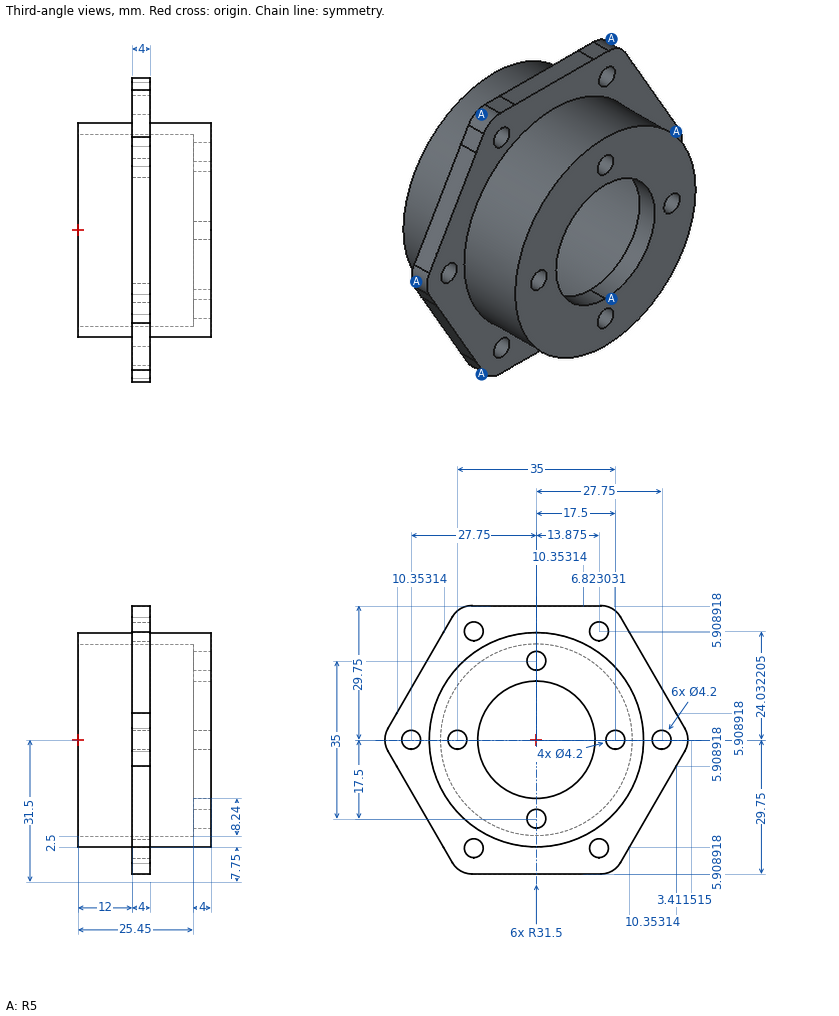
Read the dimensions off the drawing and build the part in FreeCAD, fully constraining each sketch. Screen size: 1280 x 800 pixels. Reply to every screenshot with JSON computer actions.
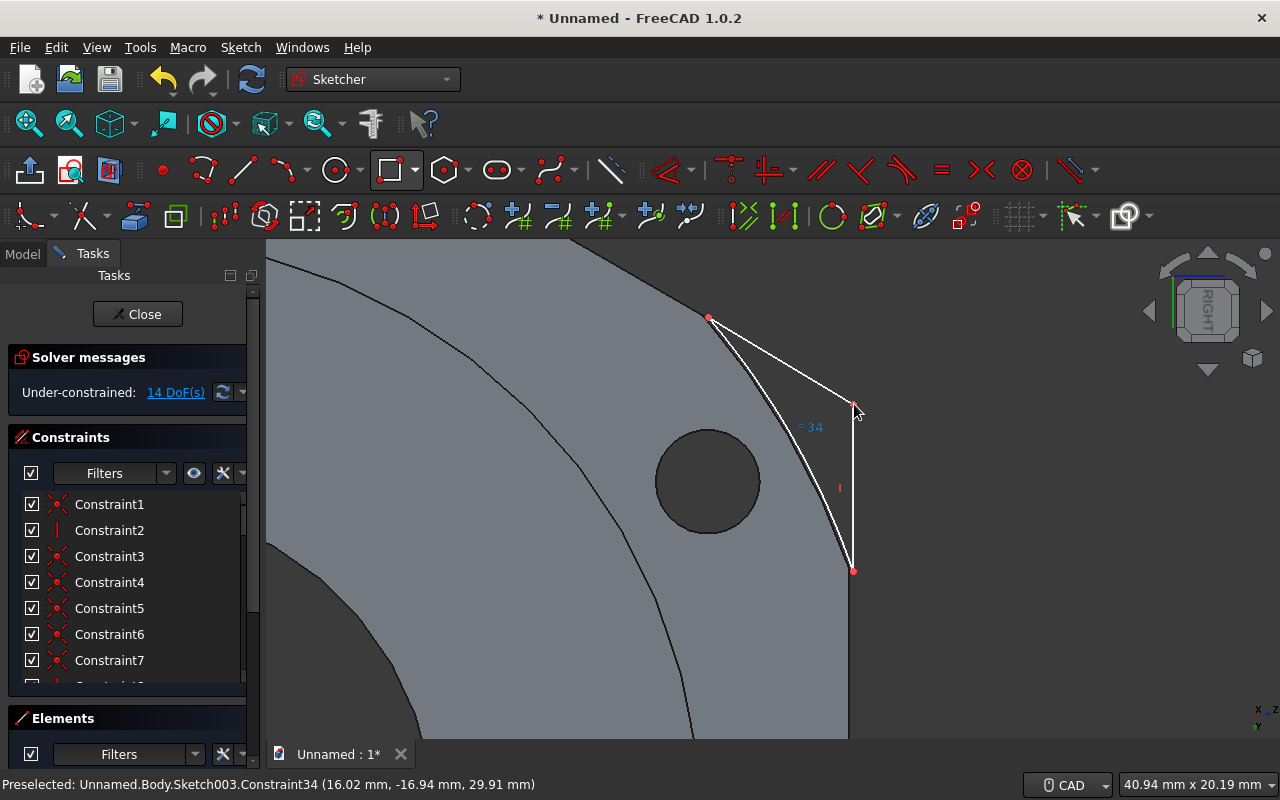
{"action": "left_click", "coordinate": [853, 404]}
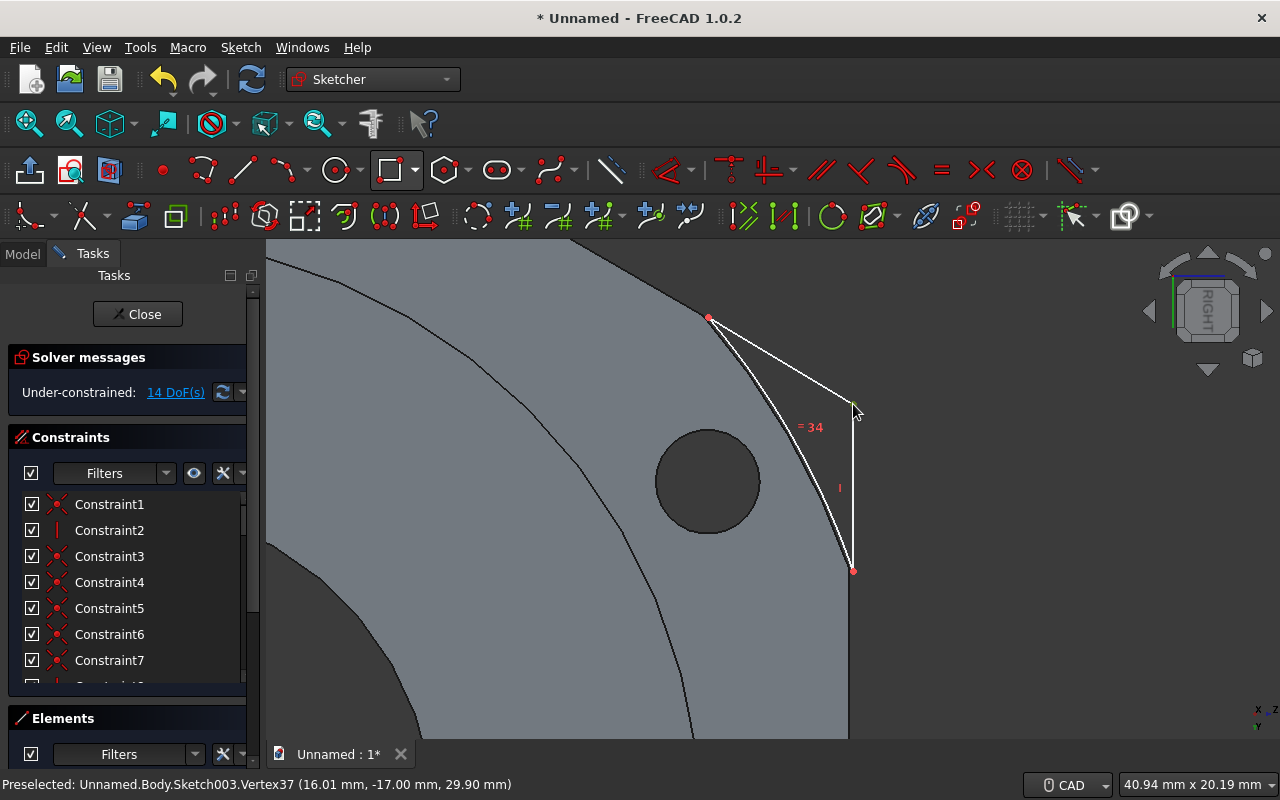
{"action": "scroll", "coordinate": [854, 404], "scroll_direction": "down", "scroll_amount": 8}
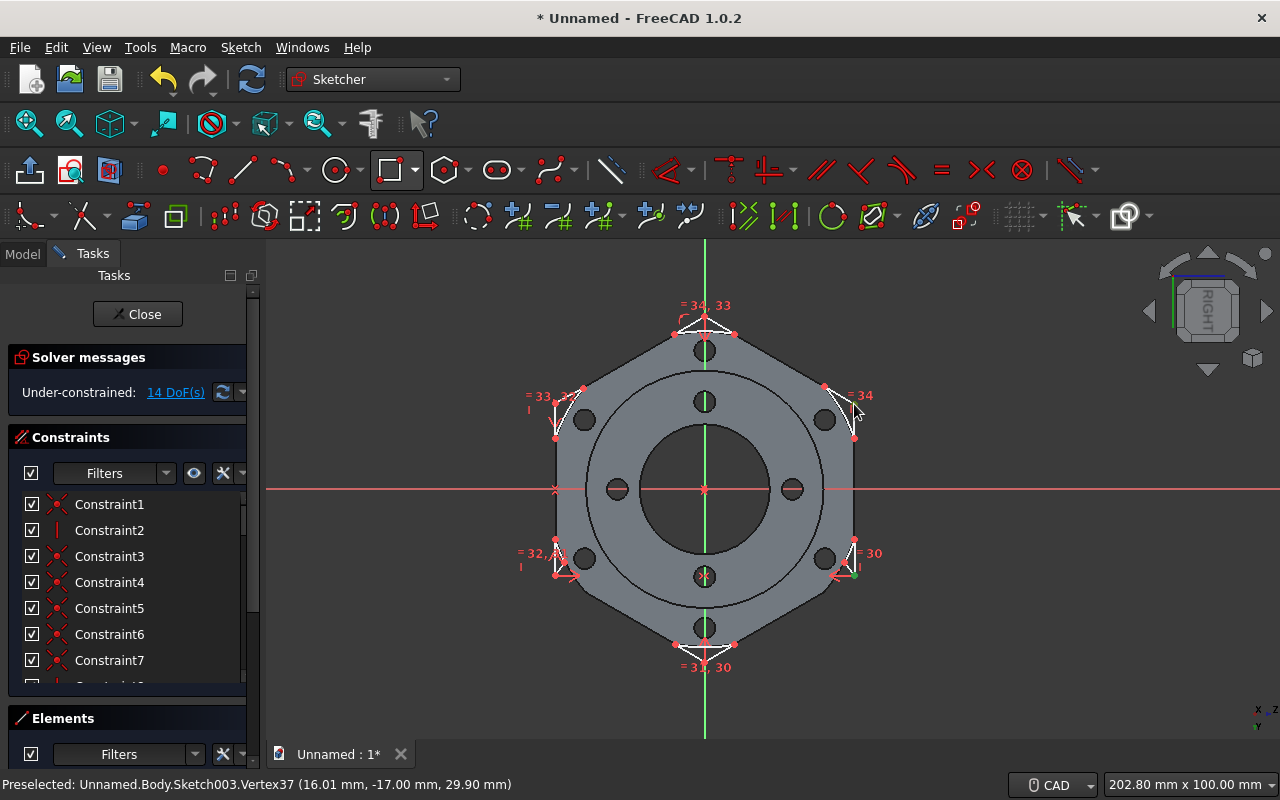
{"action": "left_click", "coordinate": [353, 489]}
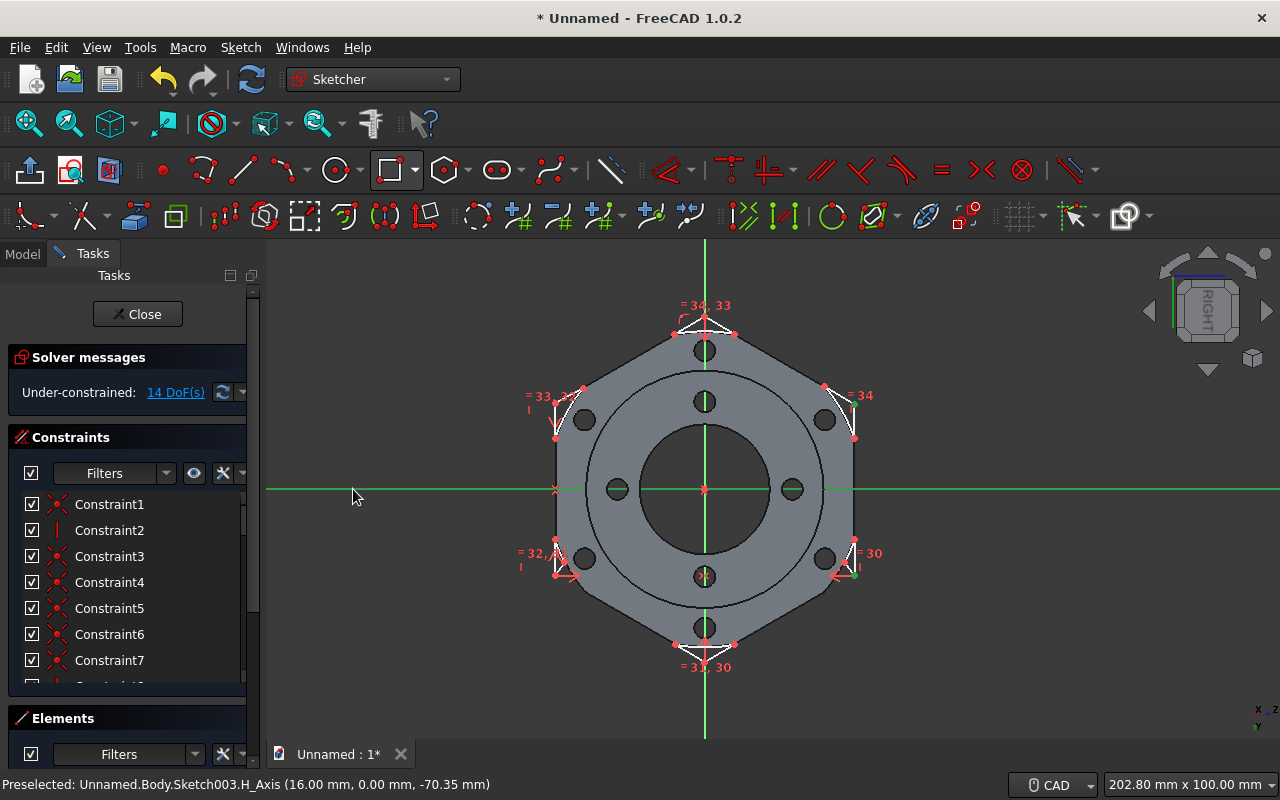
{"action": "key", "text": "s"}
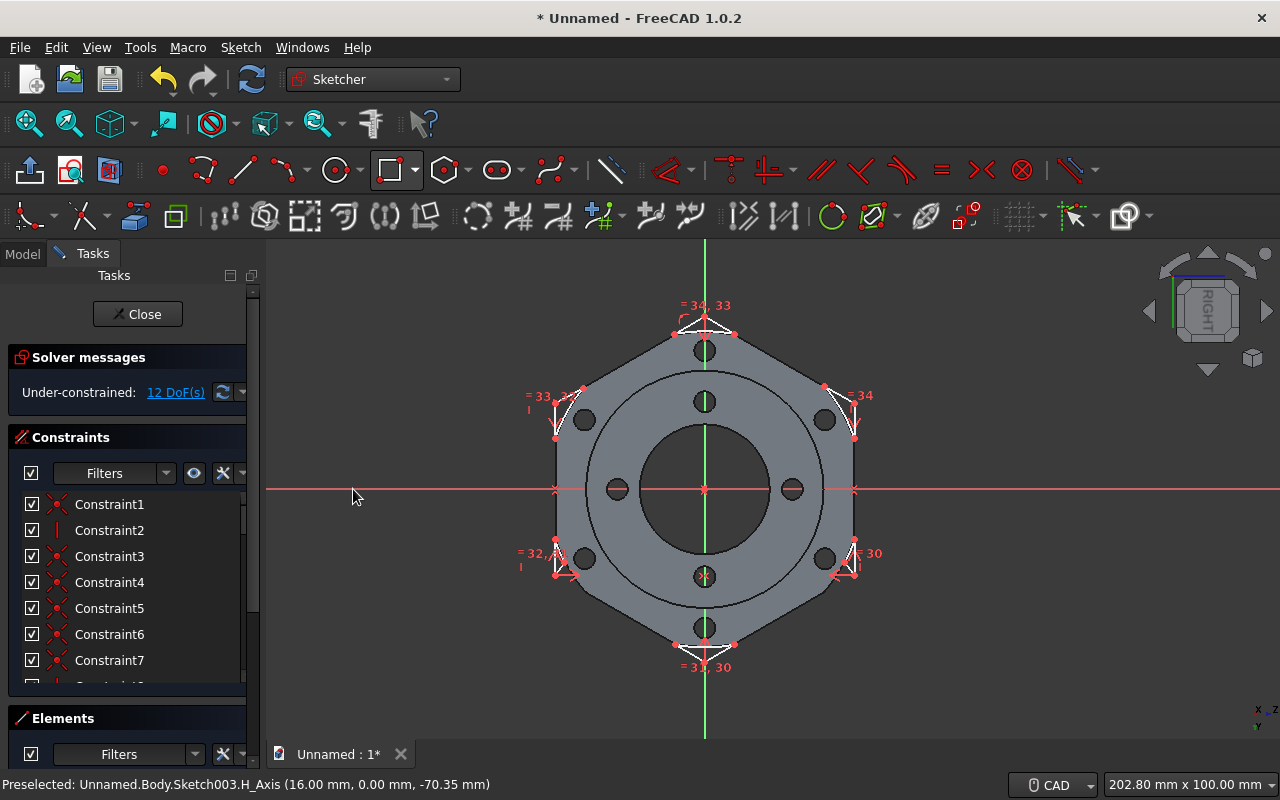
{"action": "key", "text": "d"}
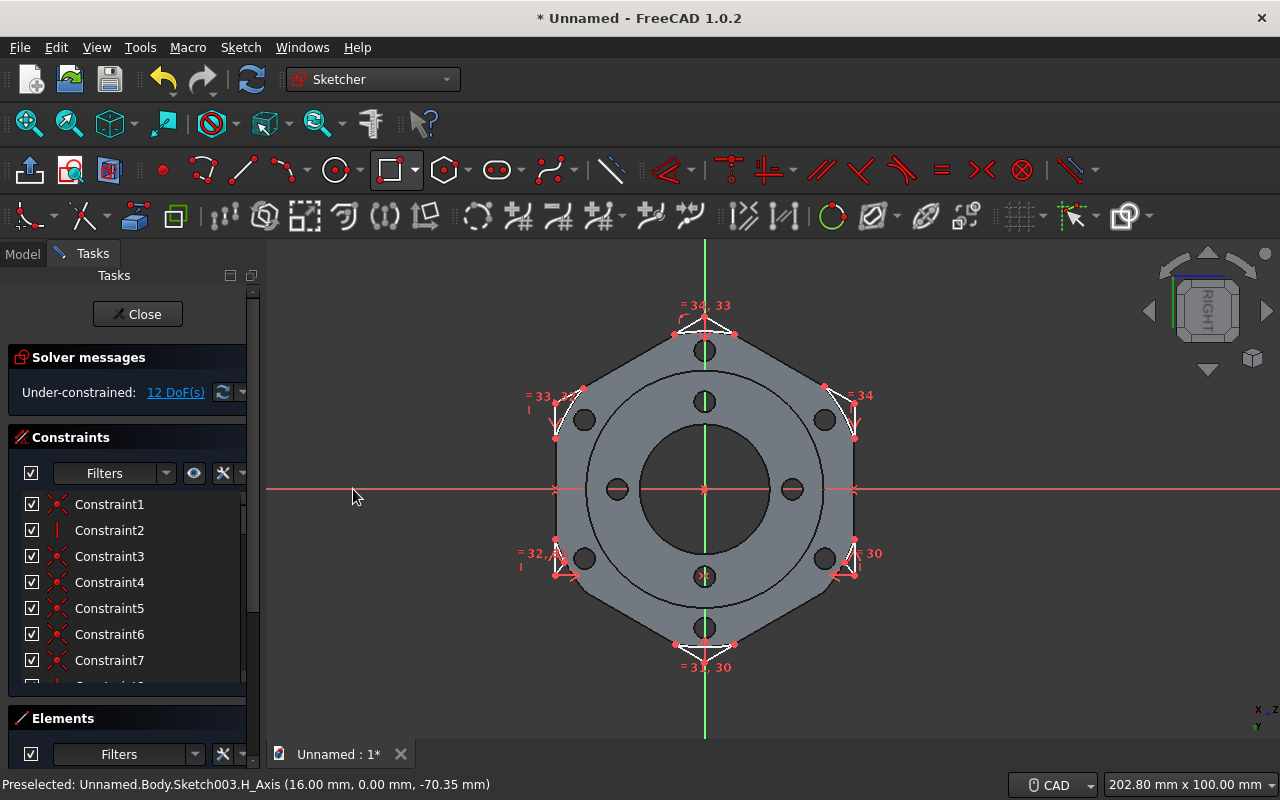
{"action": "scroll", "coordinate": [848, 556], "scroll_direction": "up", "scroll_amount": 4}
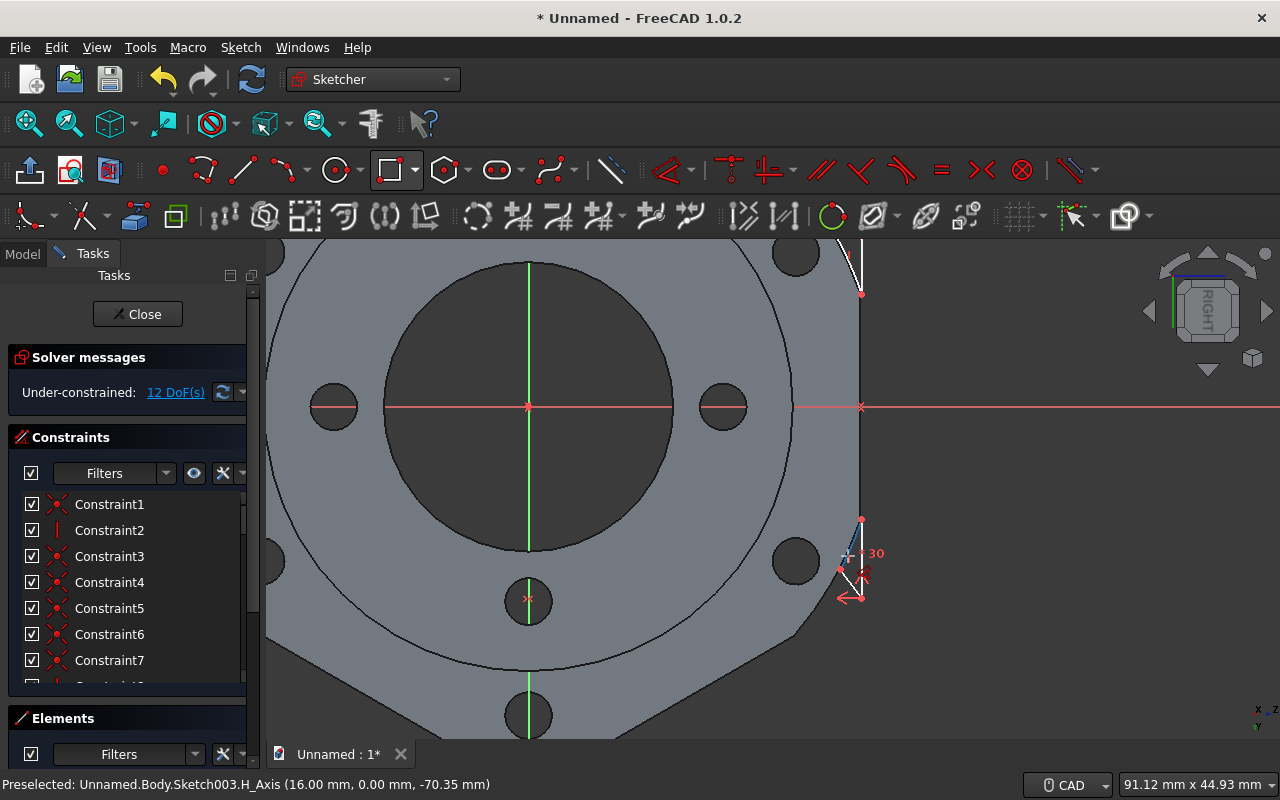
{"action": "left_click", "coordinate": [847, 555]}
{"action": "left_click", "coordinate": [876, 568]}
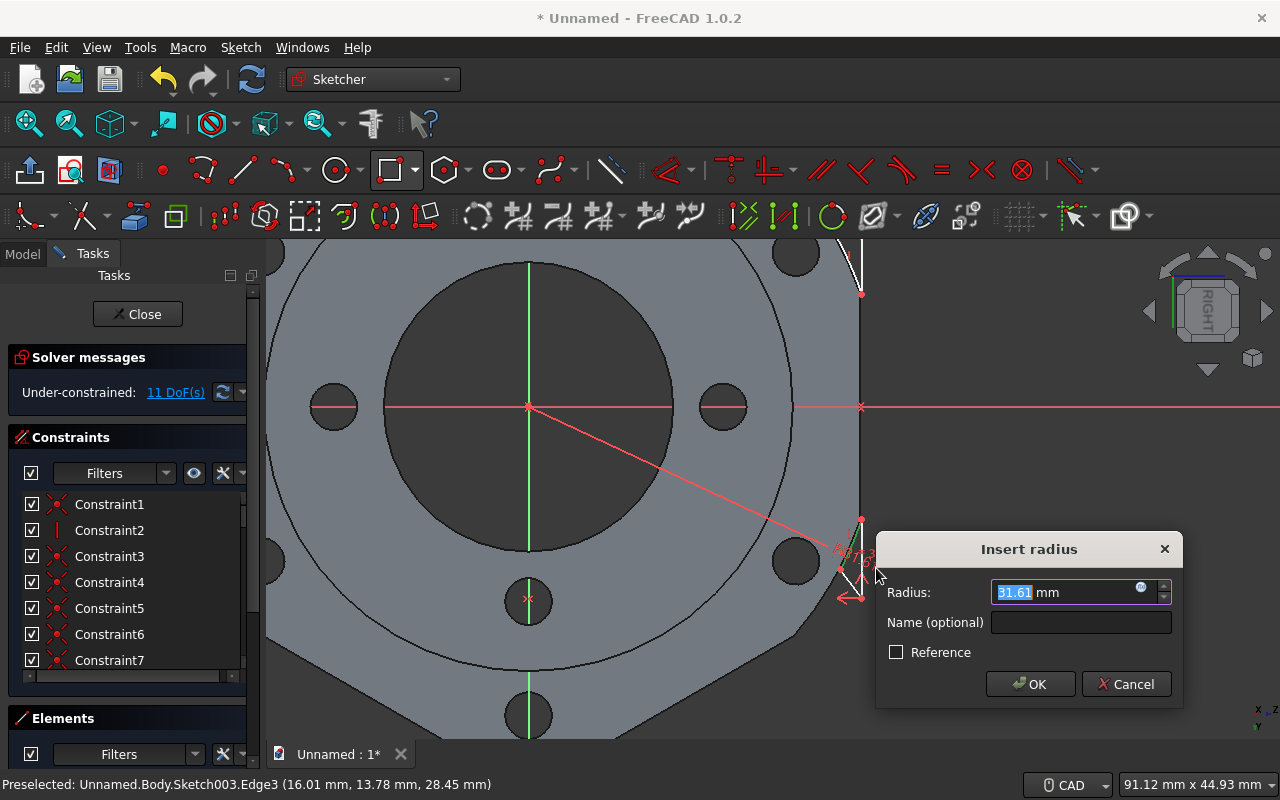
{"action": "type", "text": "31.5"}
{"action": "key", "text": "Return"}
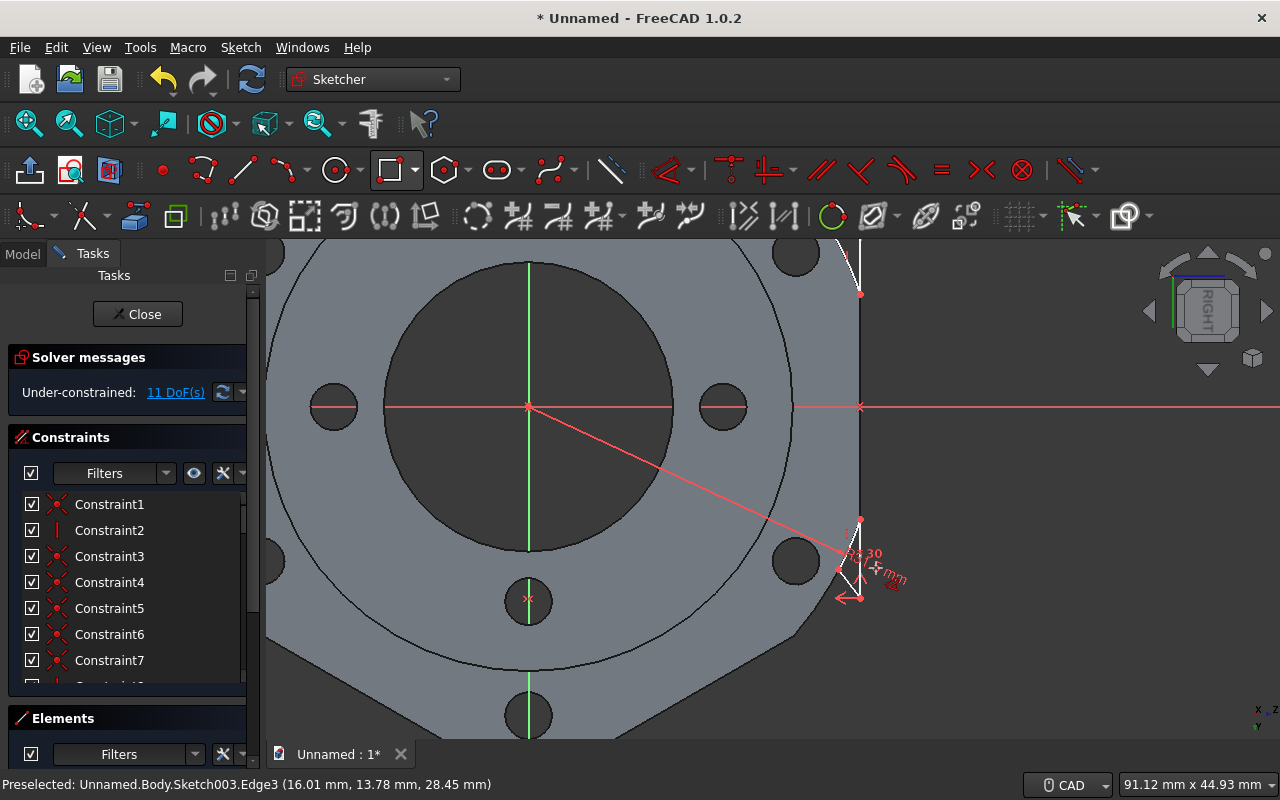
{"action": "left_click", "coordinate": [860, 575]}
{"action": "left_click", "coordinate": [894, 541]}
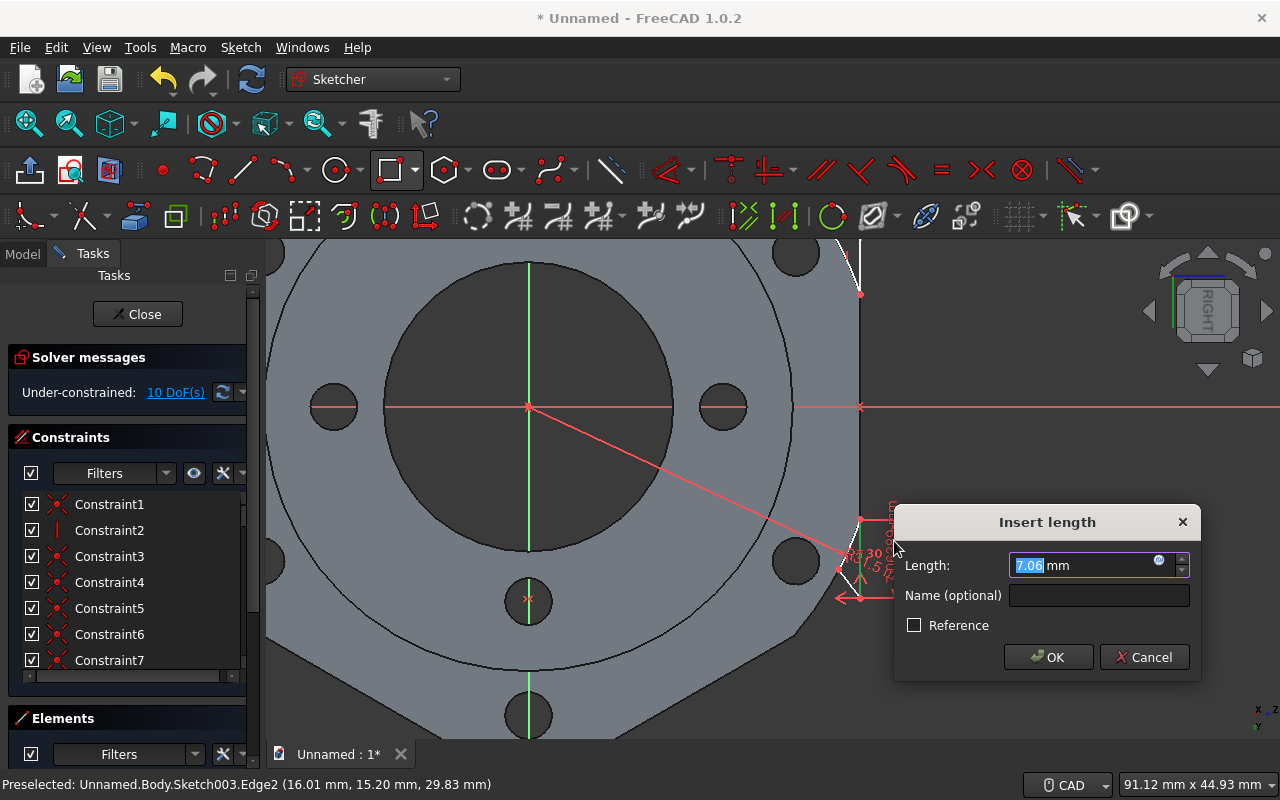
{"action": "type", "text": "6.823031"}
{"action": "key", "text": "Return"}